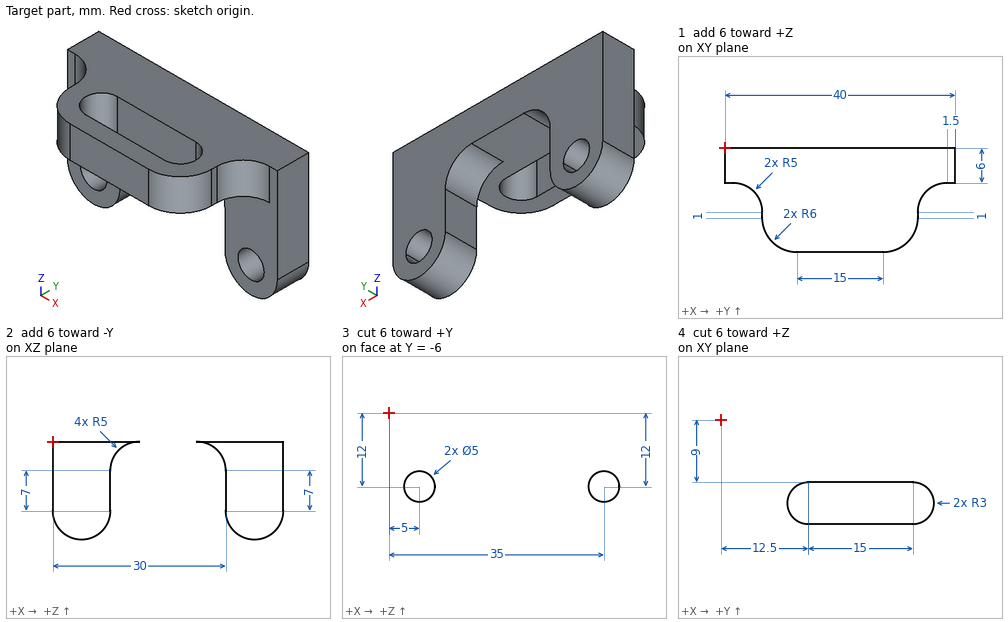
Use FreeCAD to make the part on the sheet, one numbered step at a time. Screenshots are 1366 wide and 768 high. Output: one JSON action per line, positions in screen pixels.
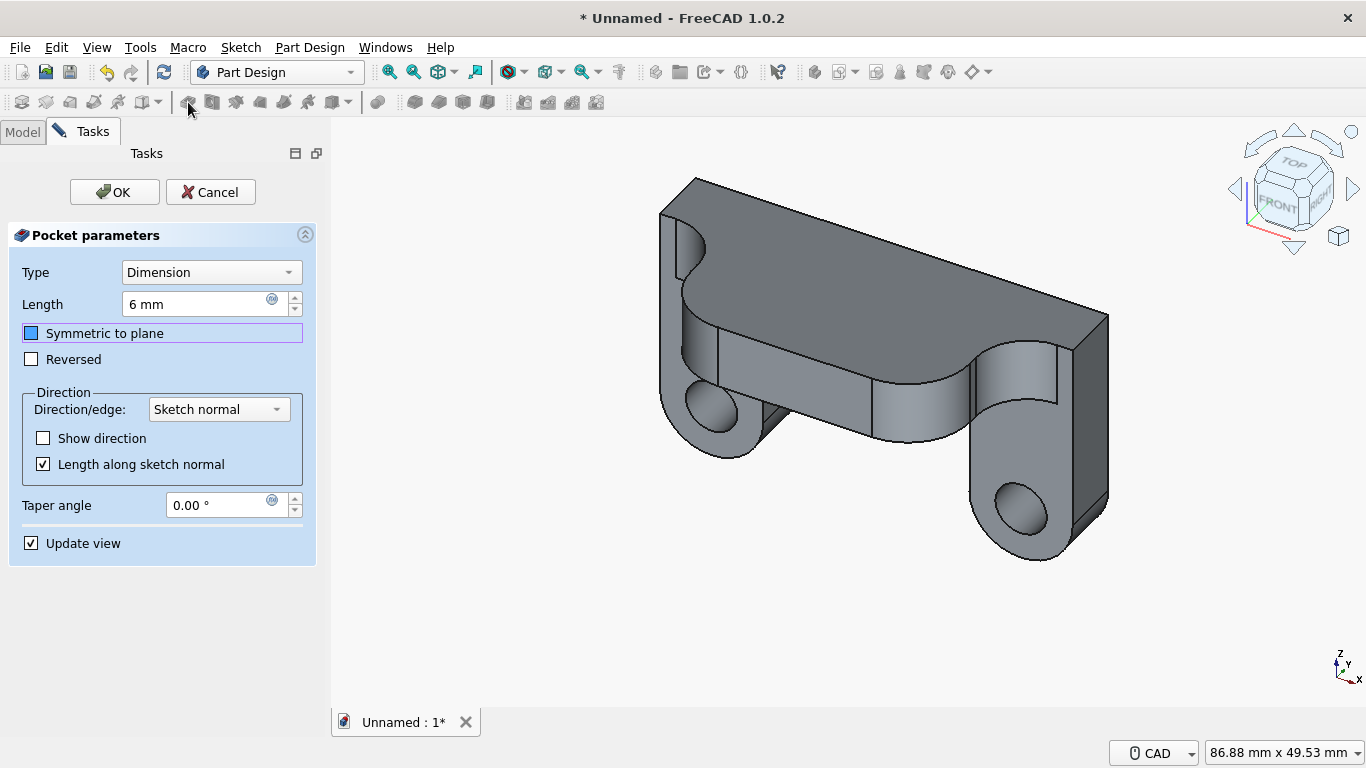
{"action": "left_click", "coordinate": [115, 192]}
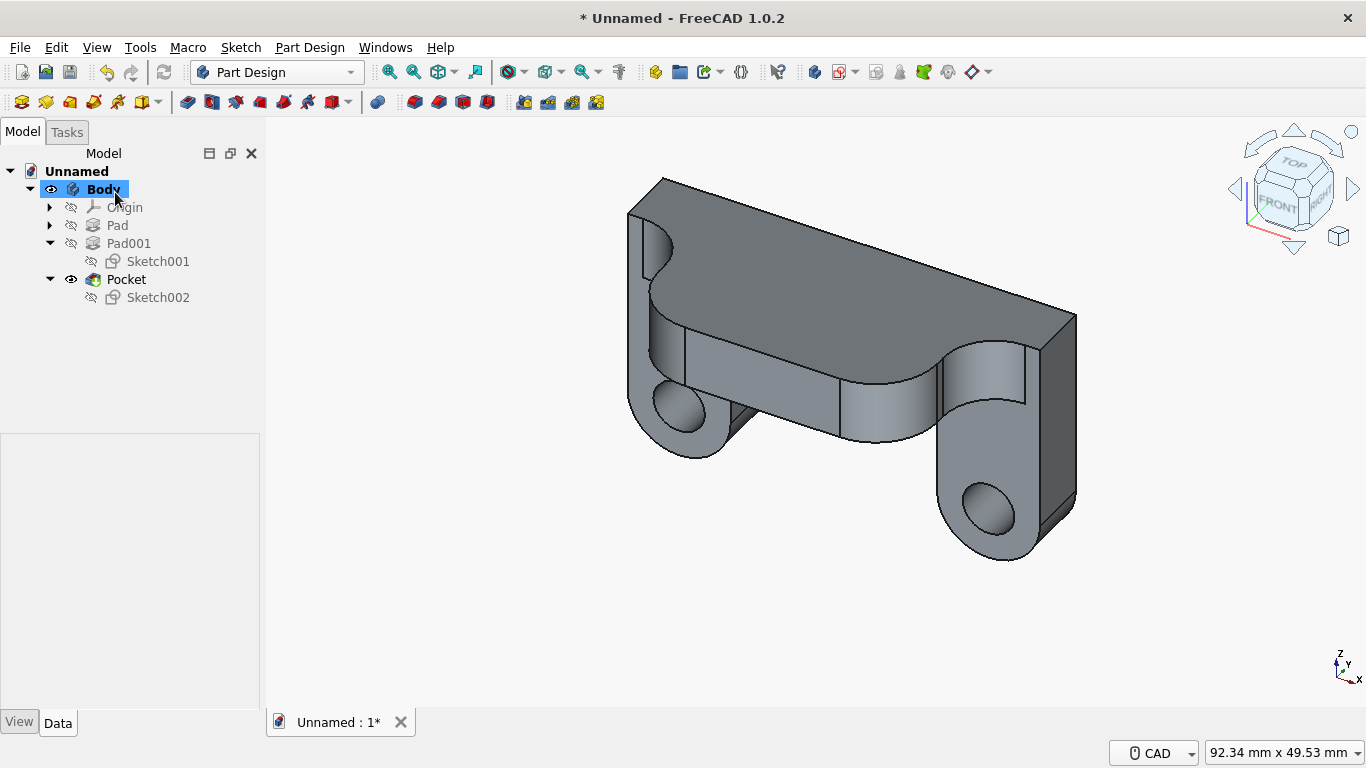
{"action": "left_click", "coordinate": [840, 72]}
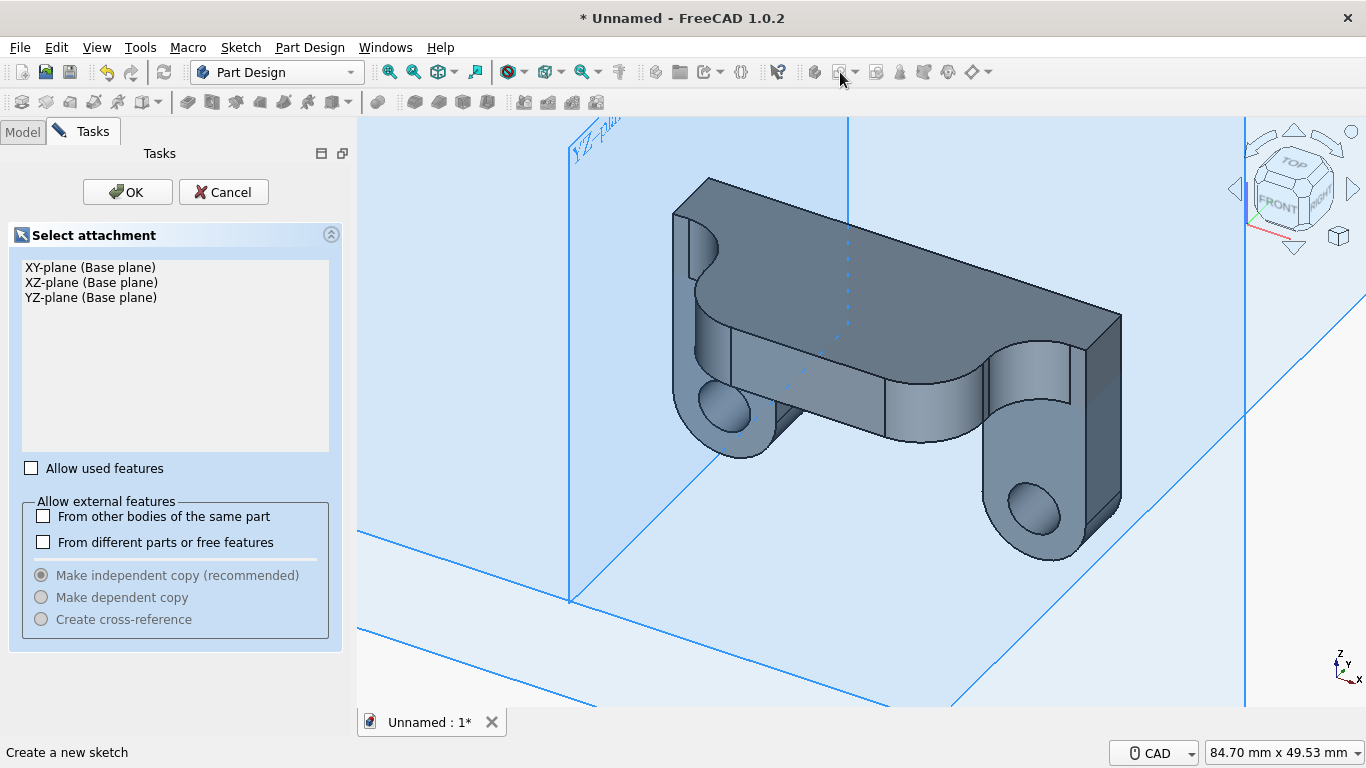
{"action": "left_click", "coordinate": [82, 268]}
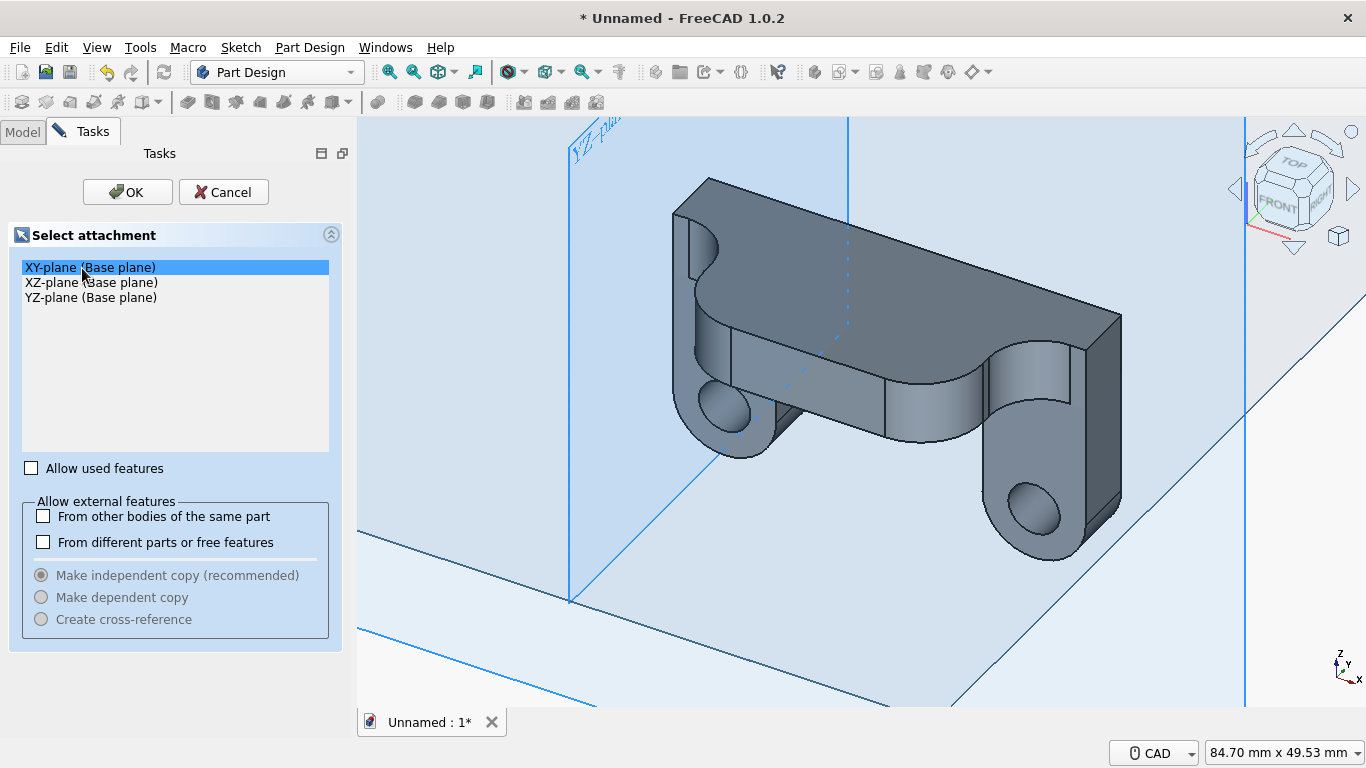
{"action": "left_click", "coordinate": [128, 192]}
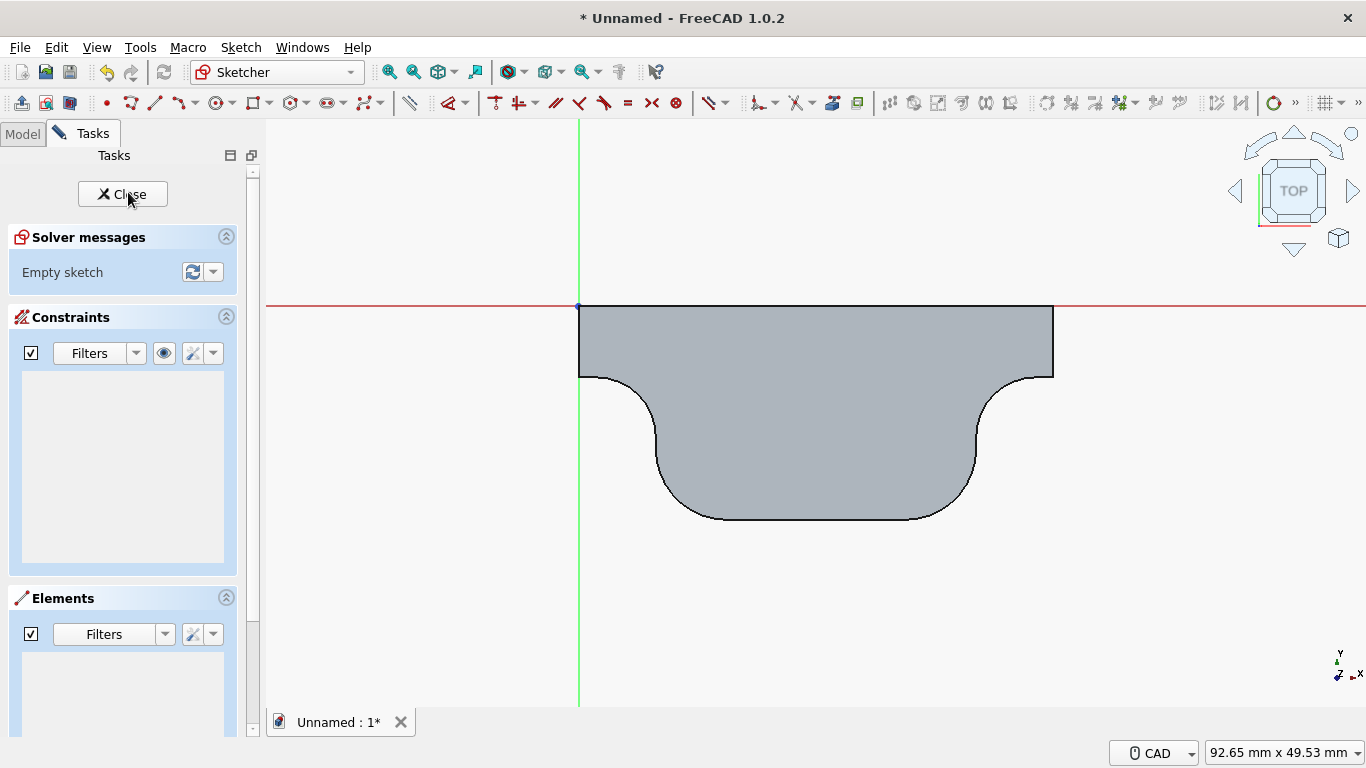
{"action": "key", "text": "q s"}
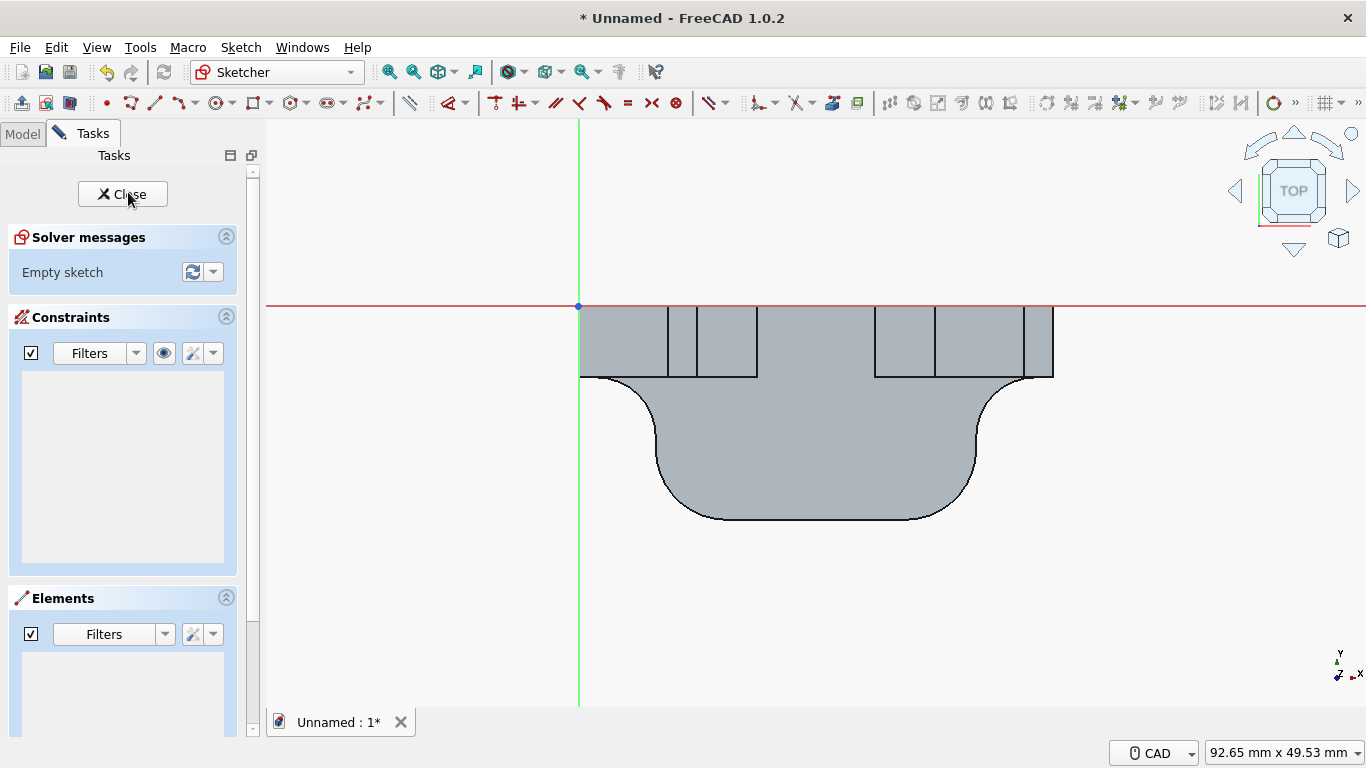
{"action": "scroll", "coordinate": [774, 374], "scroll_direction": "up", "scroll_amount": 3}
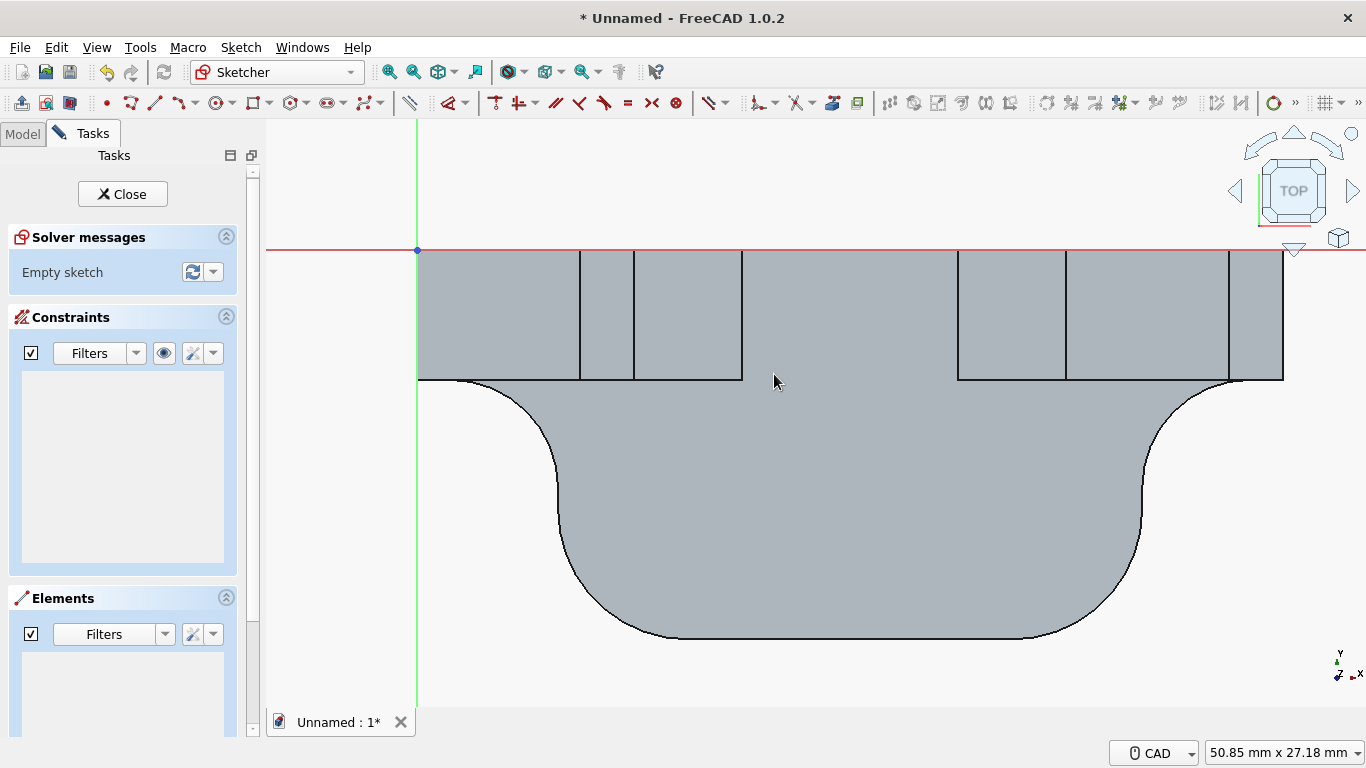
{"action": "key", "text": "g s"}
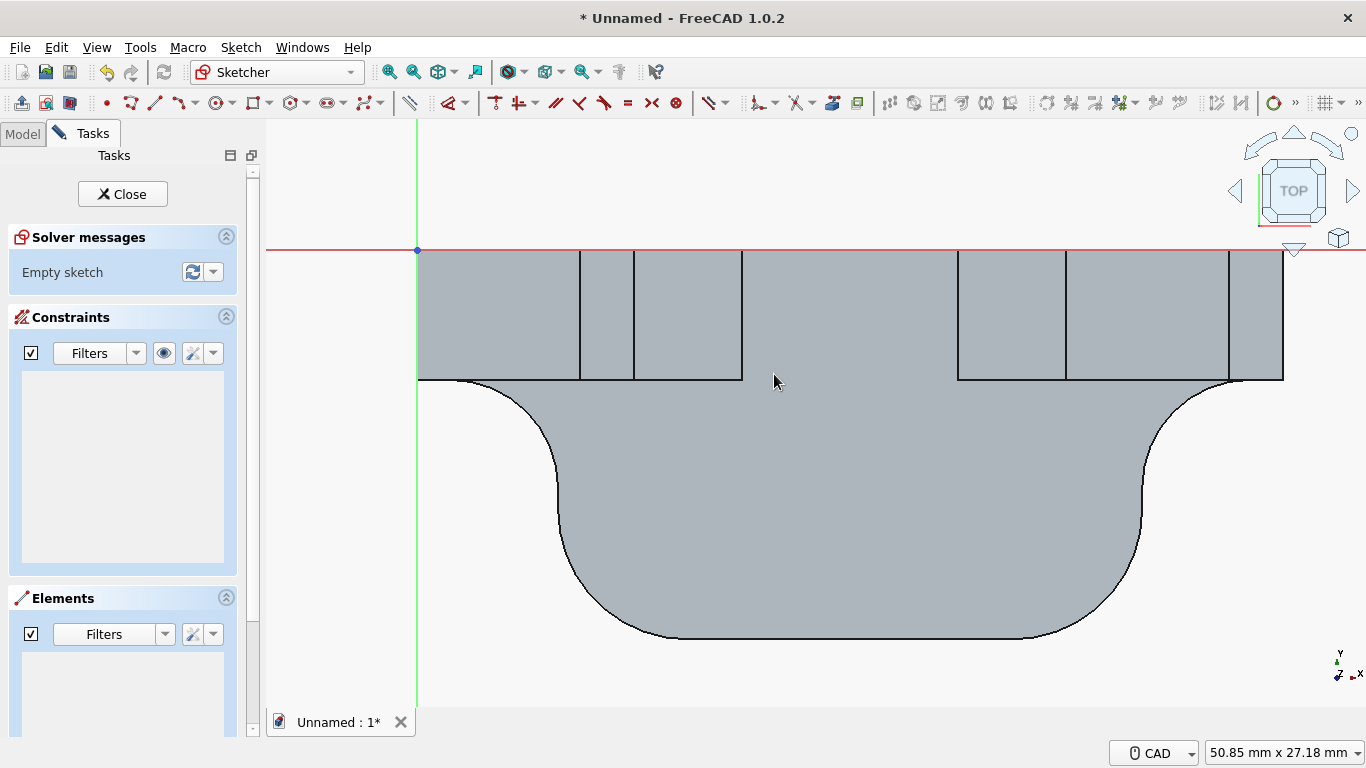
{"action": "left_click", "coordinate": [688, 510]}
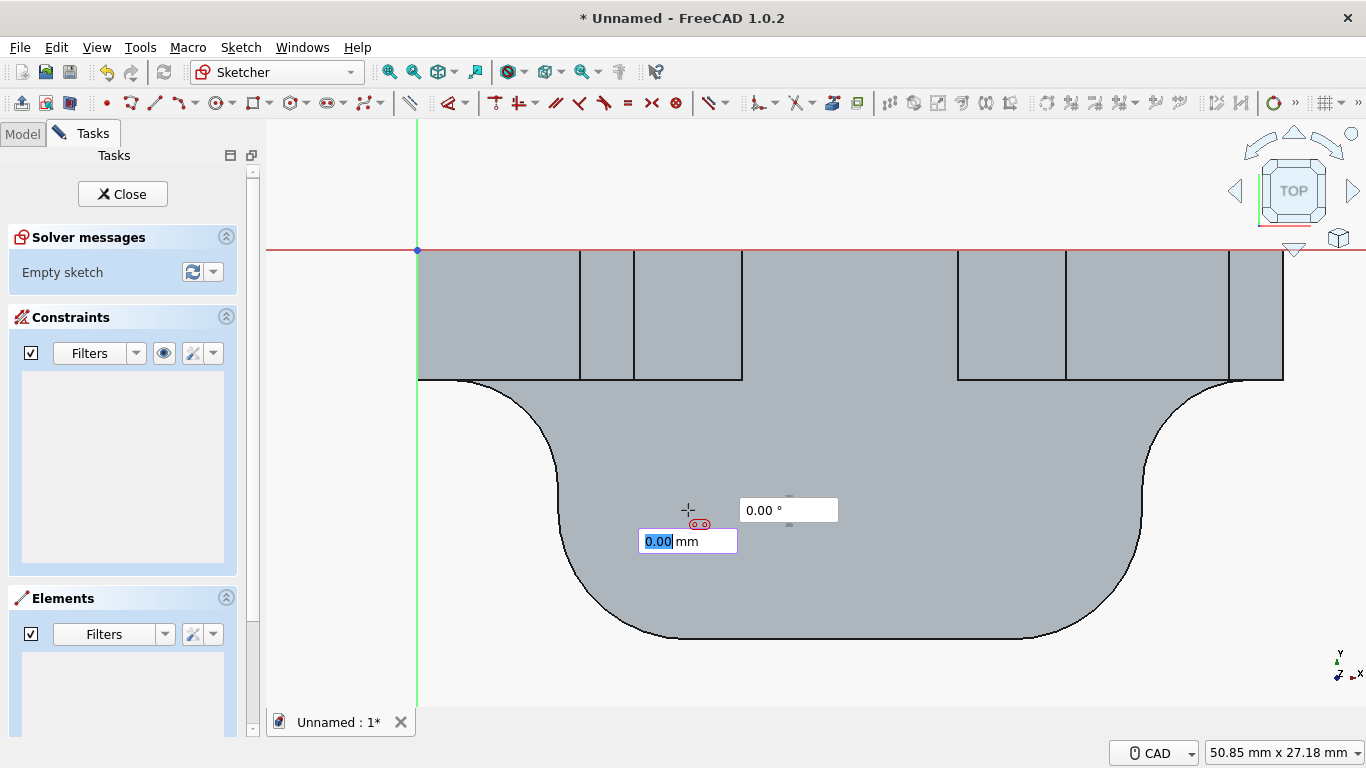
{"action": "left_click", "coordinate": [1012, 510]}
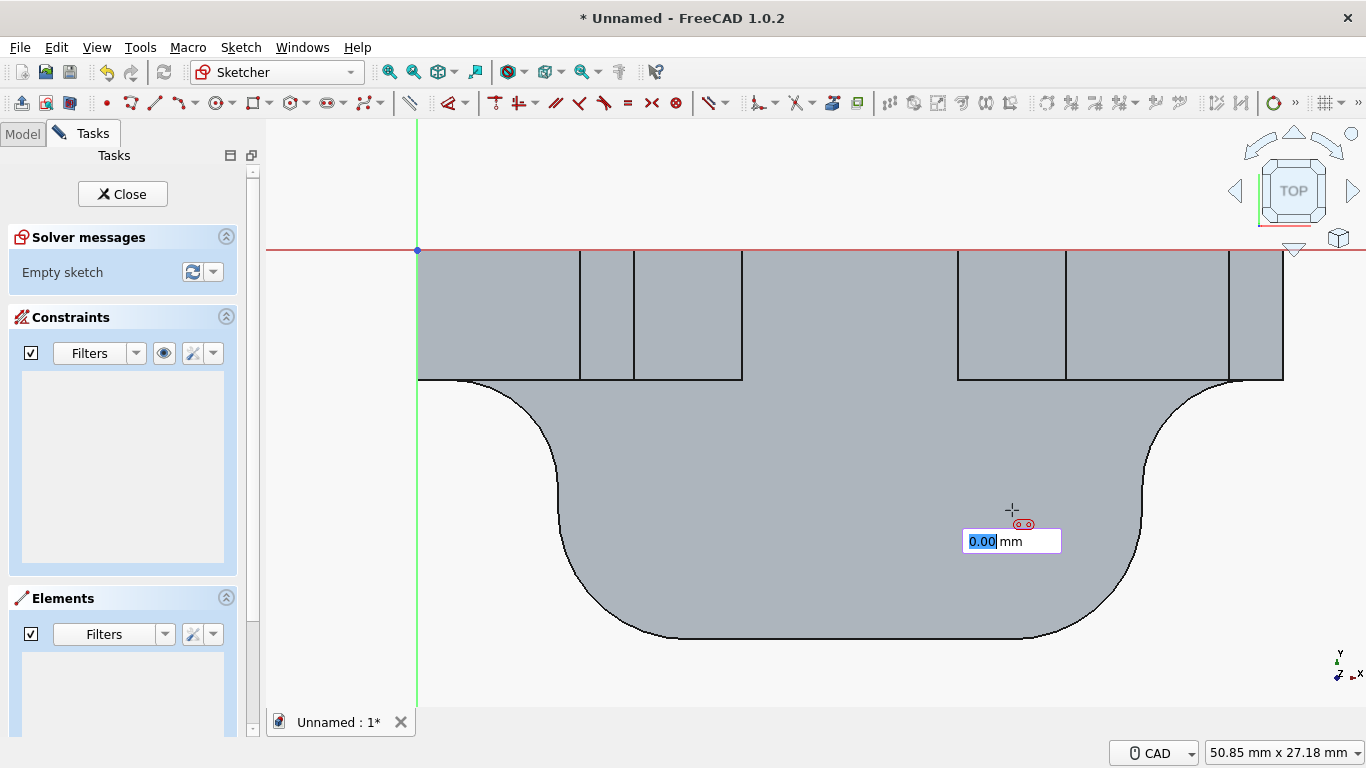
{"action": "left_click", "coordinate": [850, 445]}
{"action": "key", "text": "Escape"}